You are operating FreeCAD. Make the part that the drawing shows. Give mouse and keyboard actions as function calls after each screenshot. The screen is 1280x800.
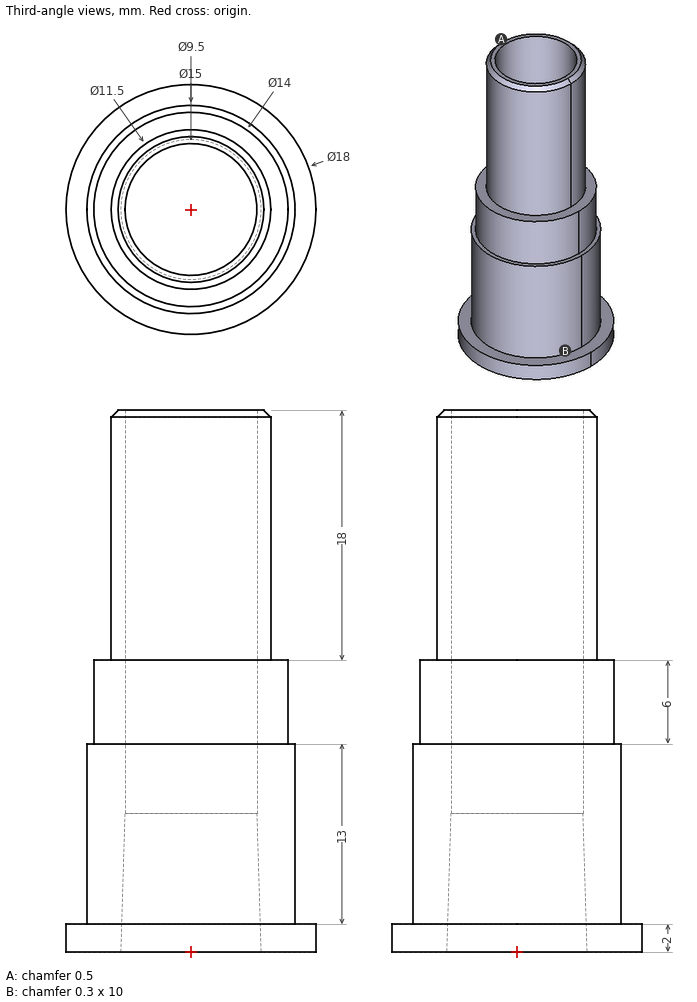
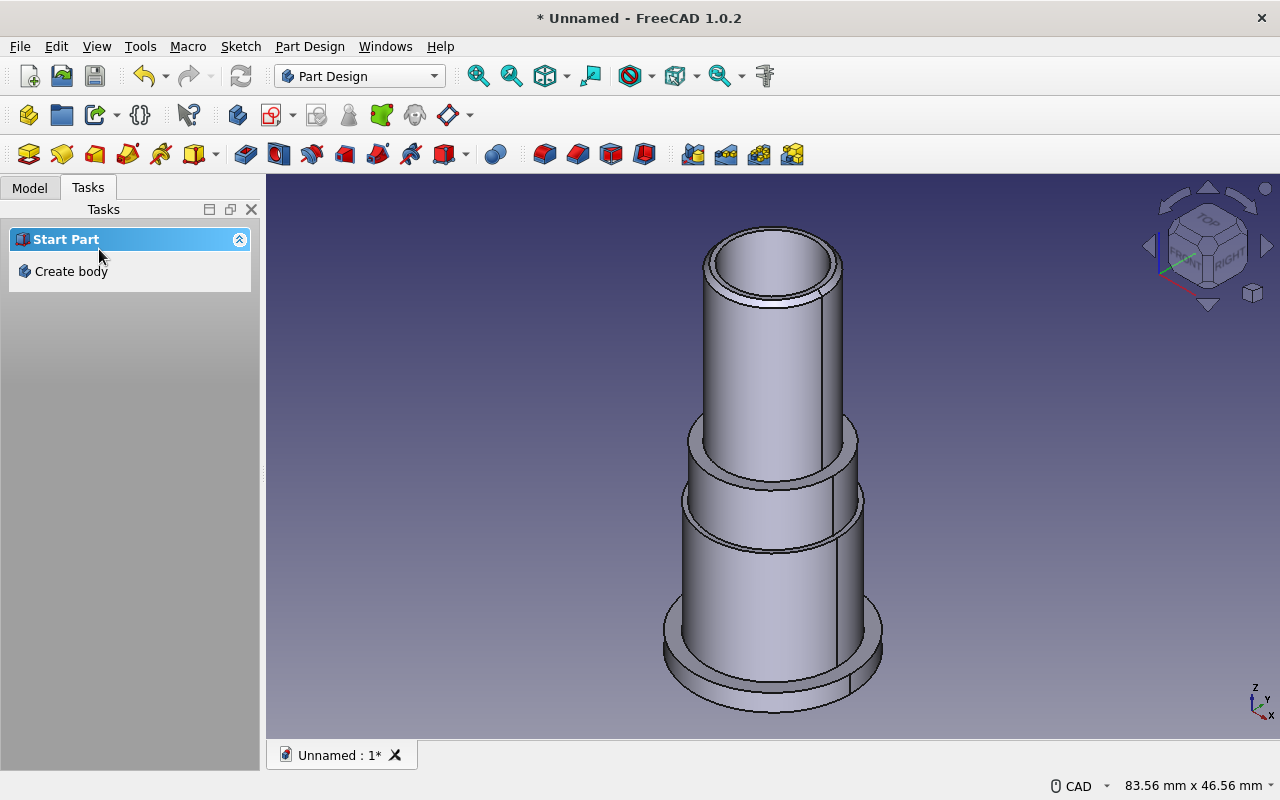
click(479, 76)